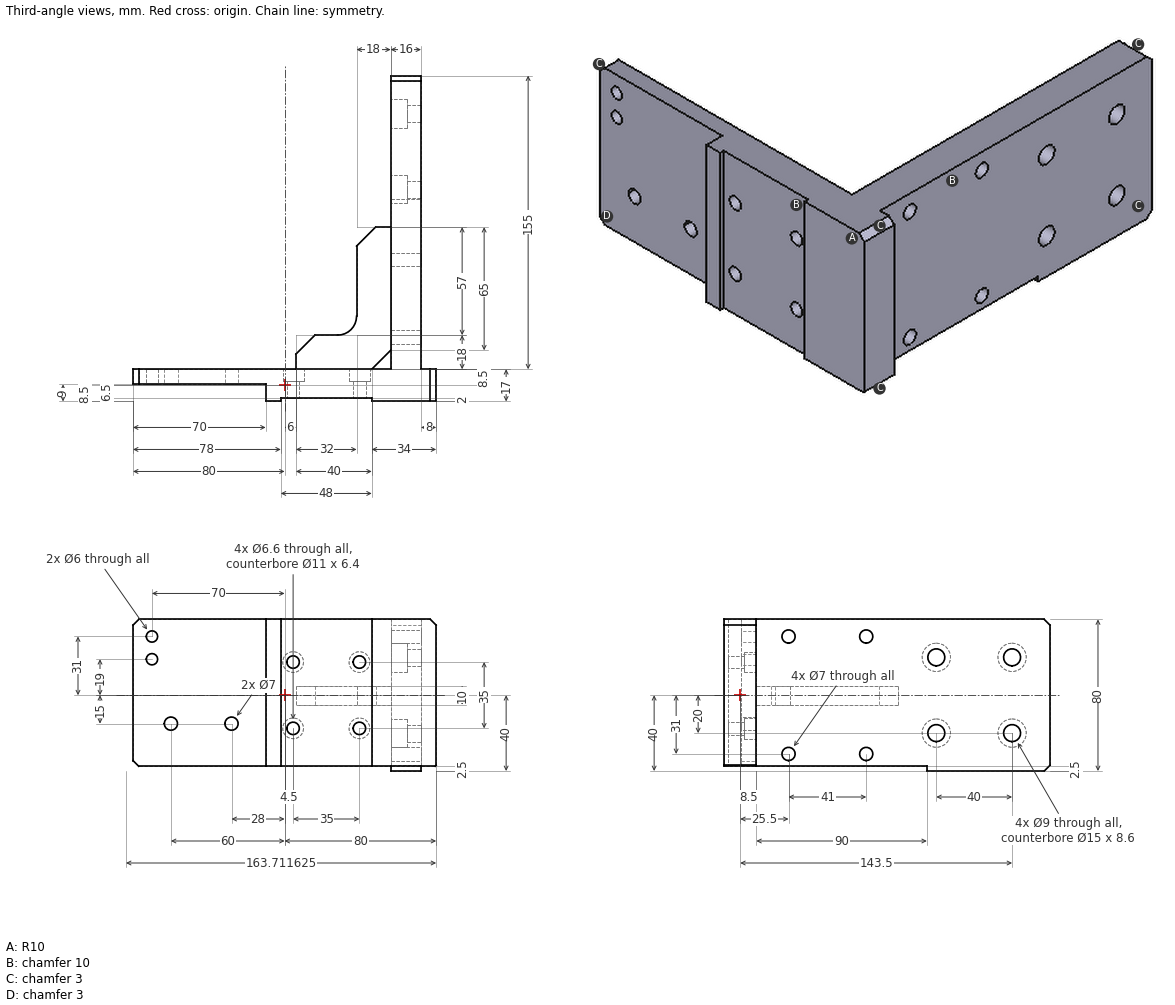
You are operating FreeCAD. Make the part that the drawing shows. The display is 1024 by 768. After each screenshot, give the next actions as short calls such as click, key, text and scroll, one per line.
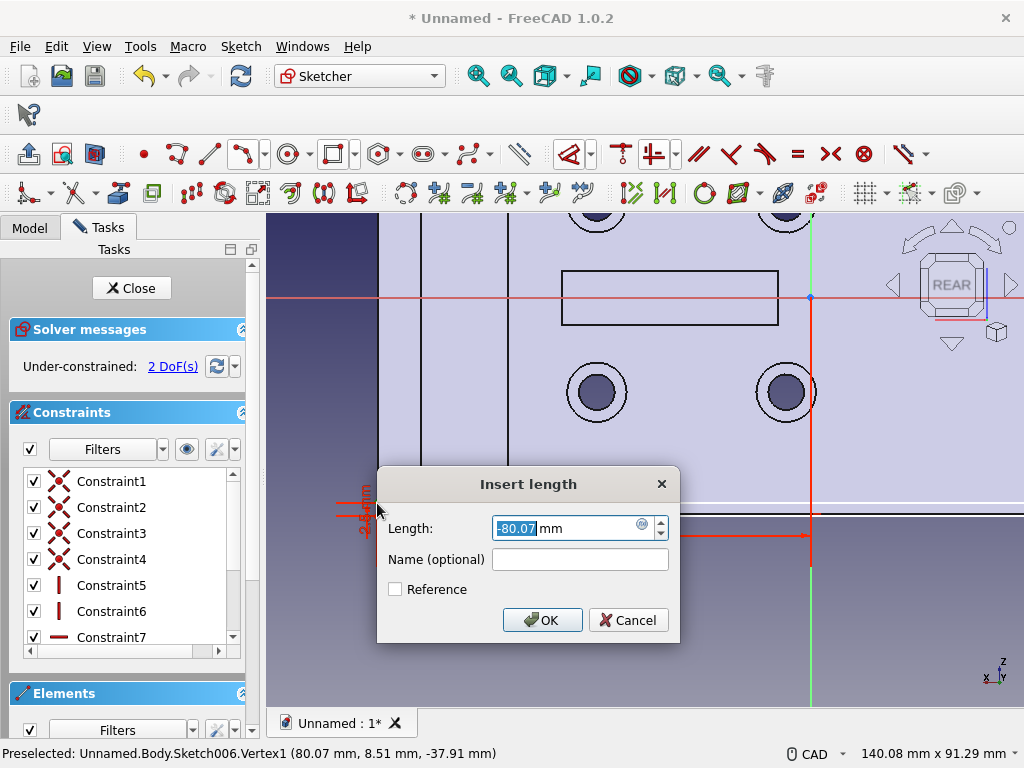
text(-80)
key(Return)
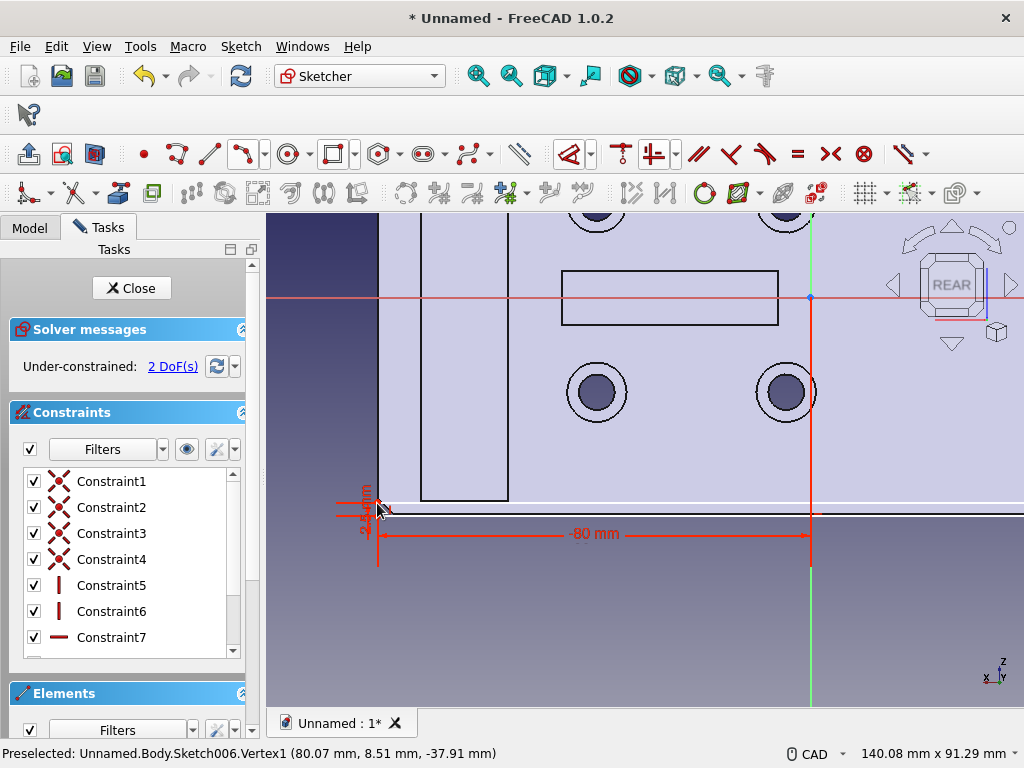
click(378, 516)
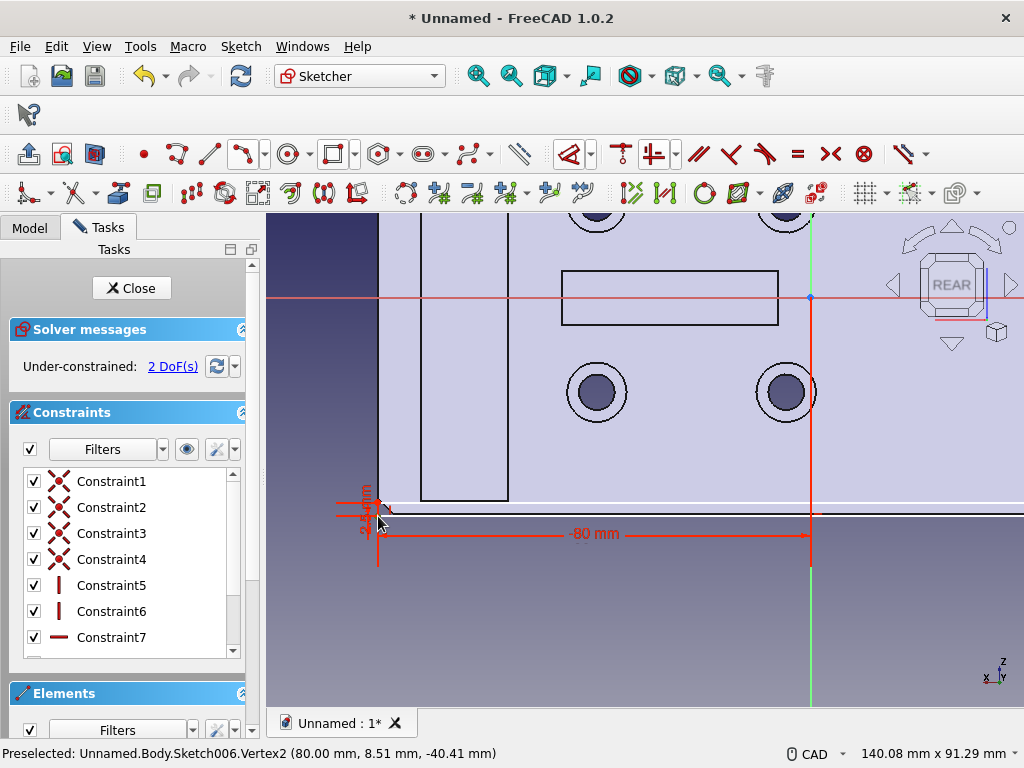
key(i)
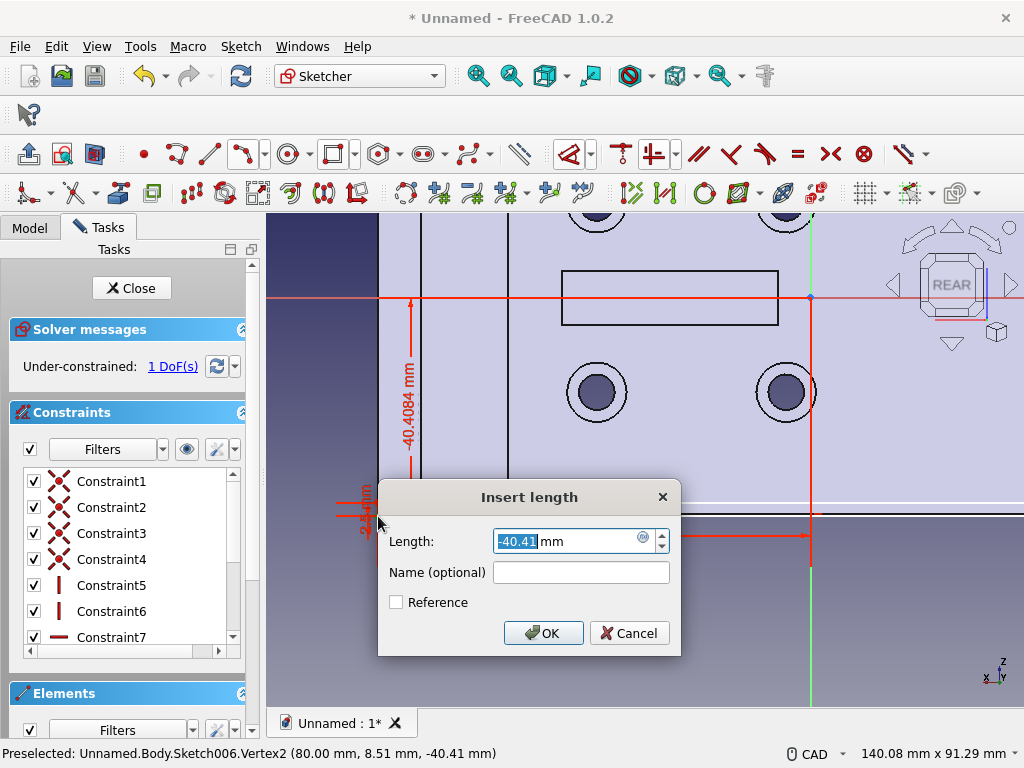
text(-40)
key(Return)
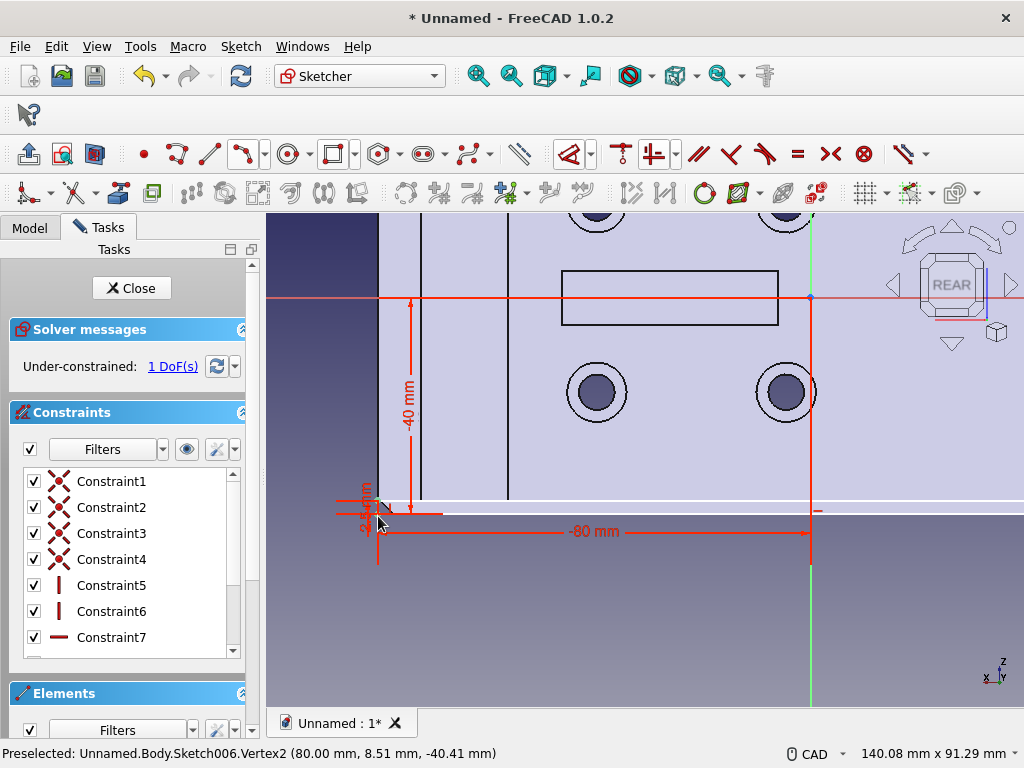
click(643, 514)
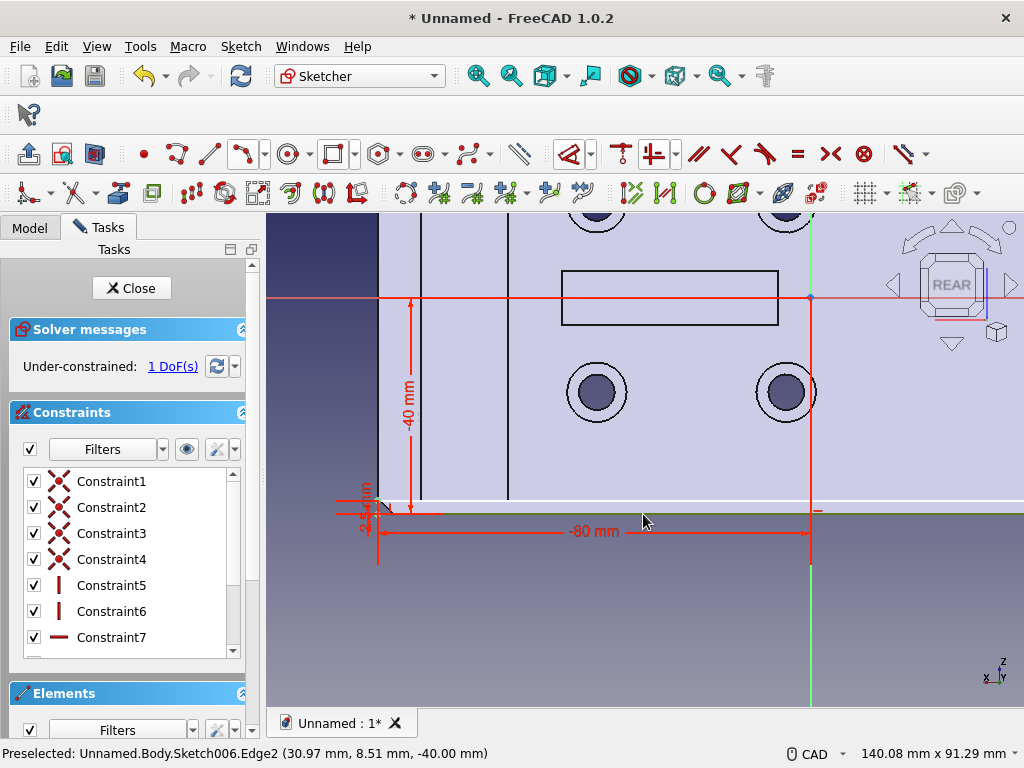
key(l)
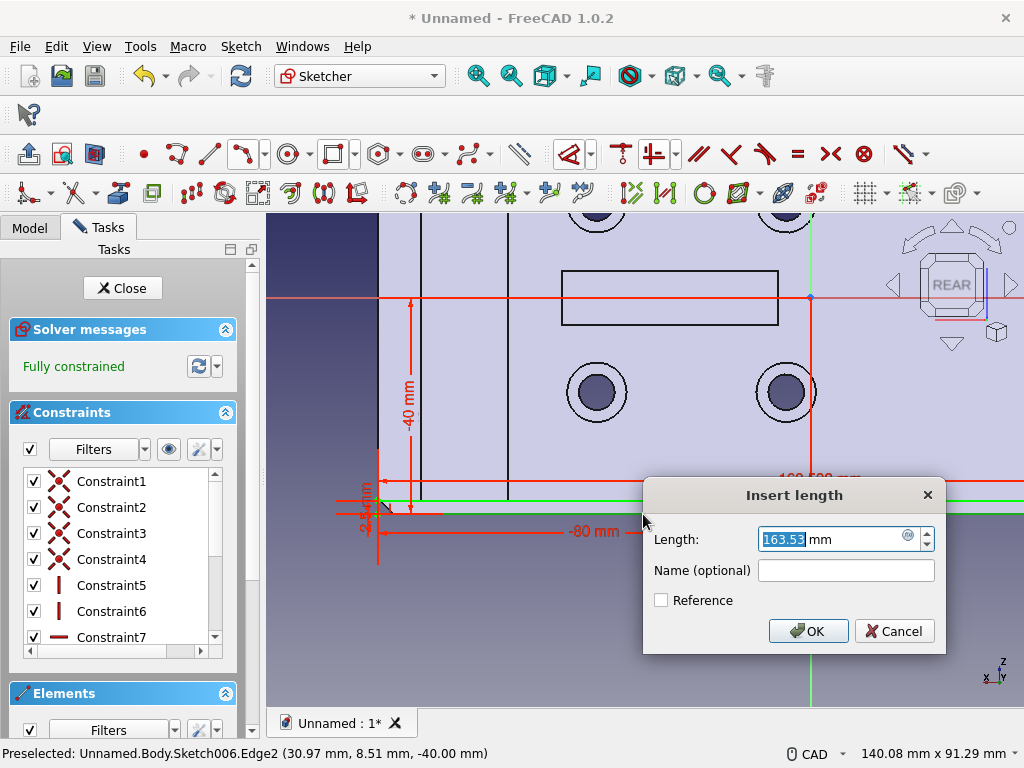
text(163.711625)
key(Return)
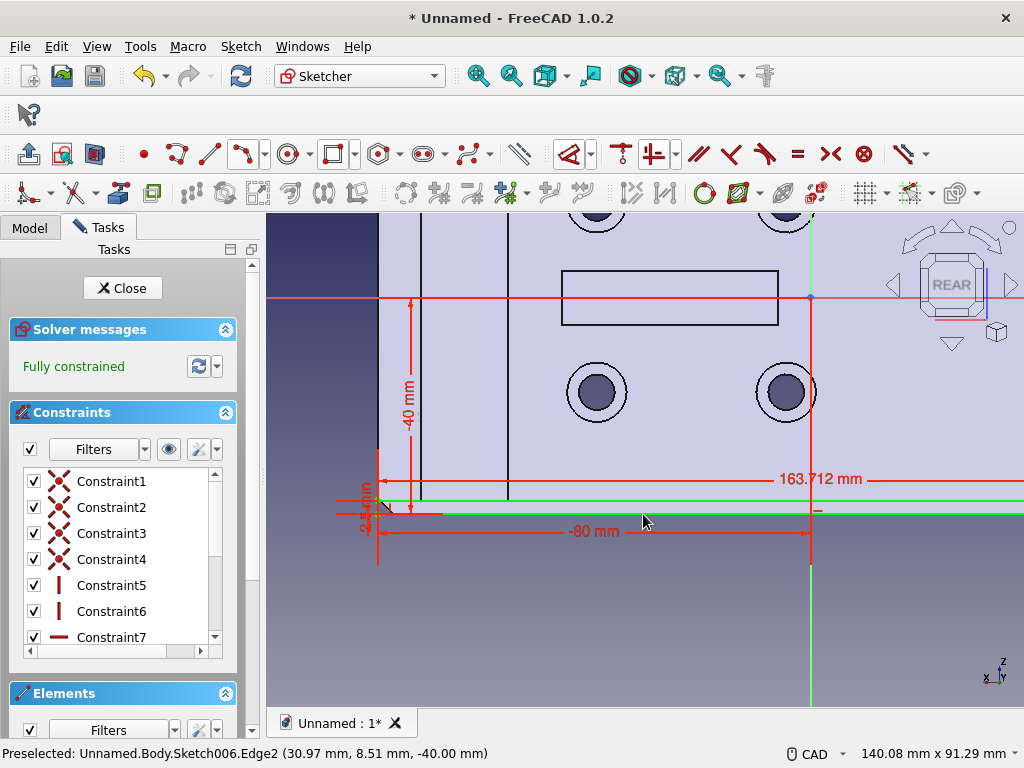
click(123, 288)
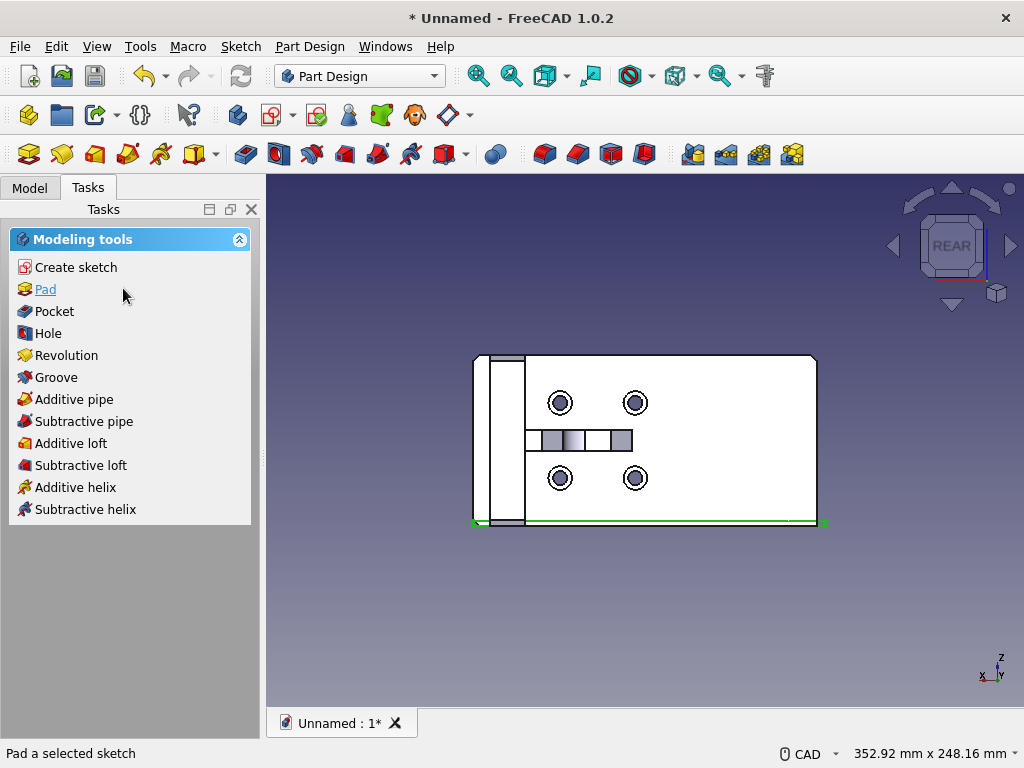
click(246, 154)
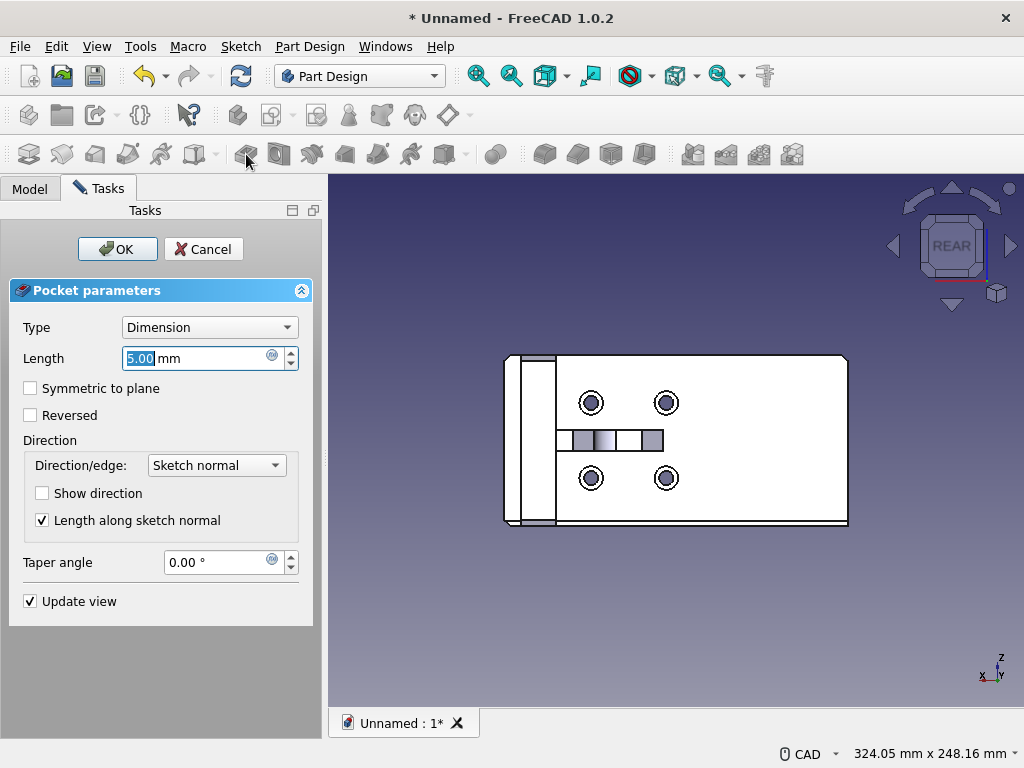
click(210, 328)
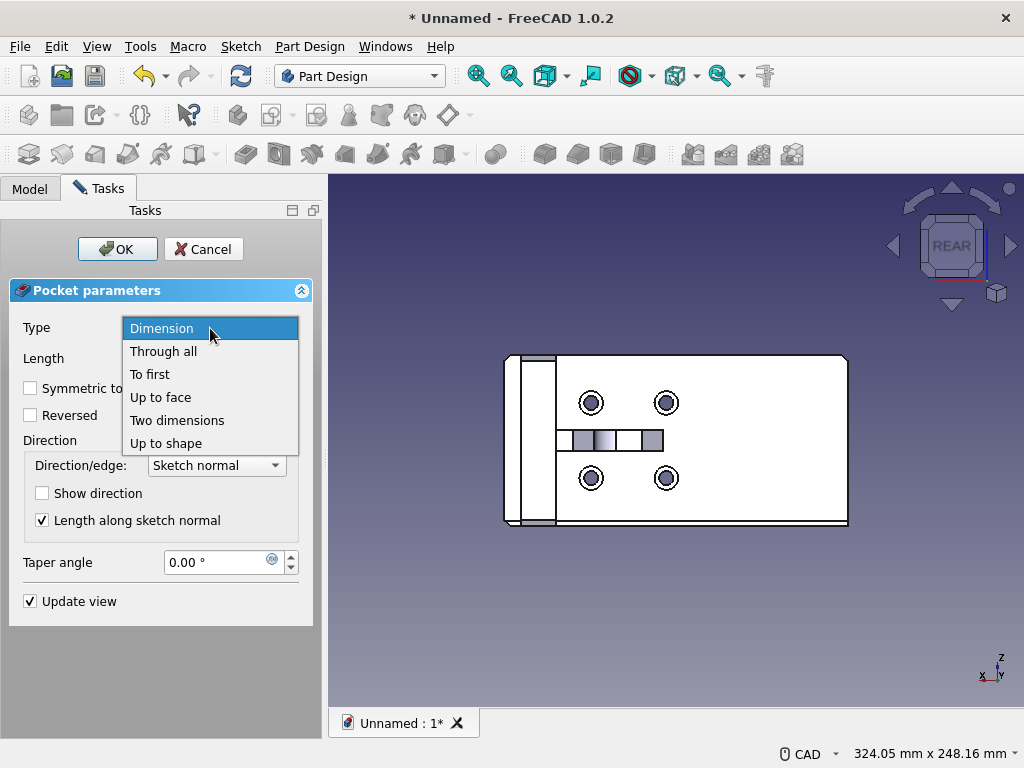
click(208, 352)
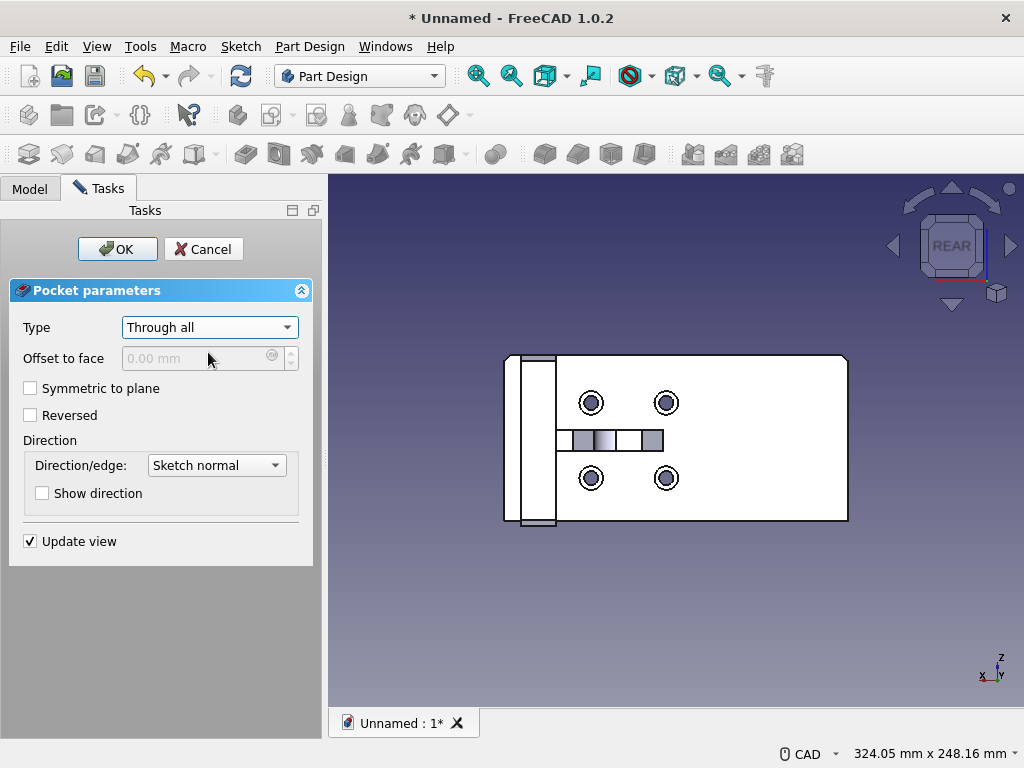
click(118, 249)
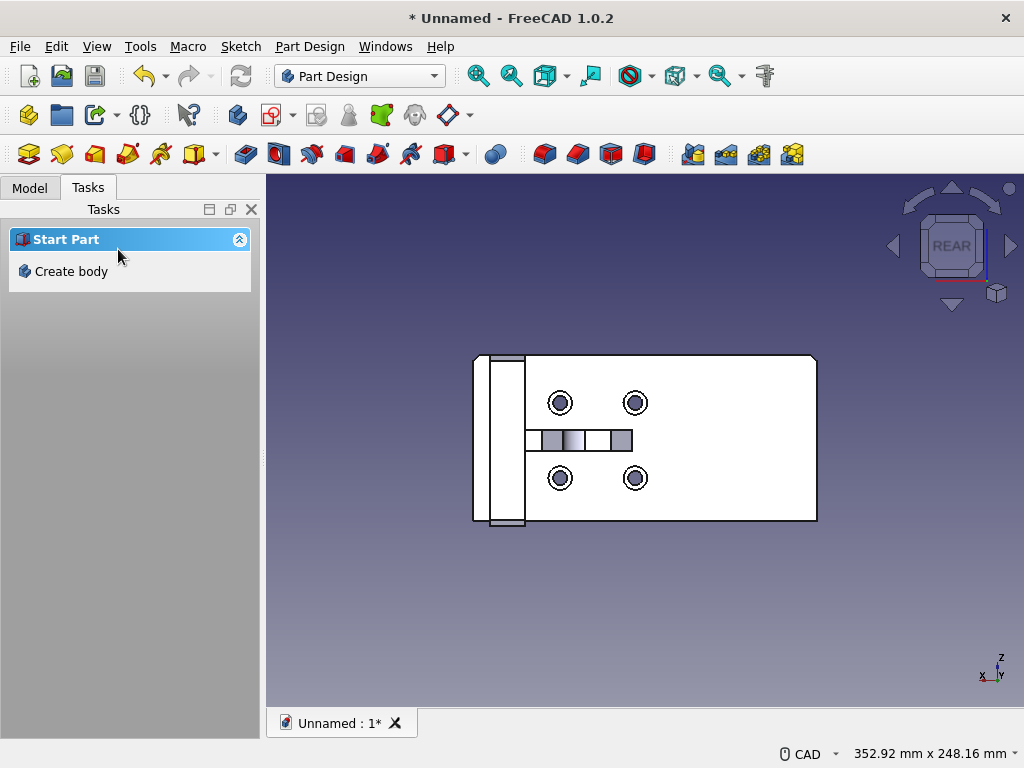
key(5)